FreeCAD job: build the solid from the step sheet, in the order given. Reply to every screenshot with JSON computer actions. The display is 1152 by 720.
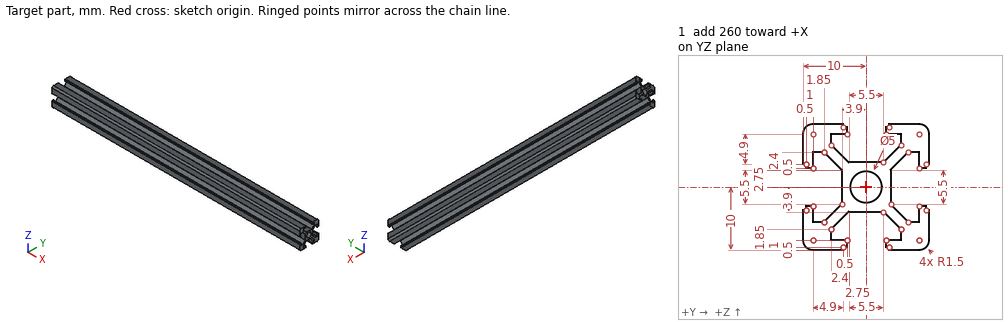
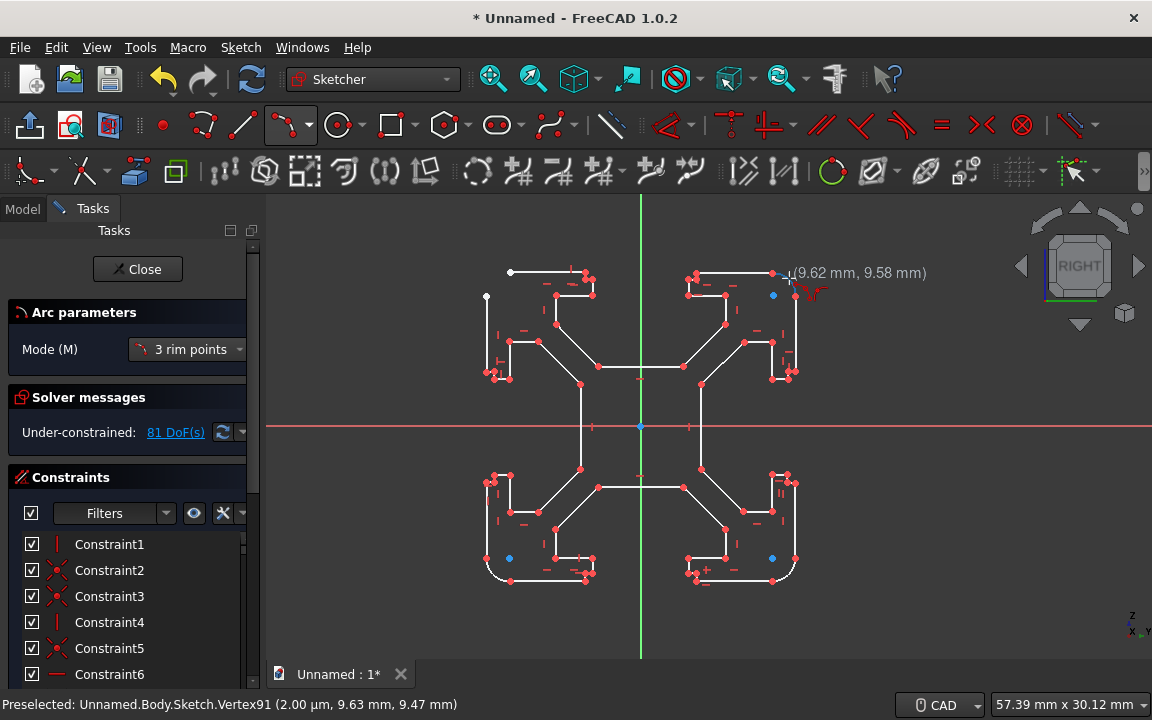
{"action": "left_click", "coordinate": [510, 272]}
{"action": "left_click", "coordinate": [487, 296]}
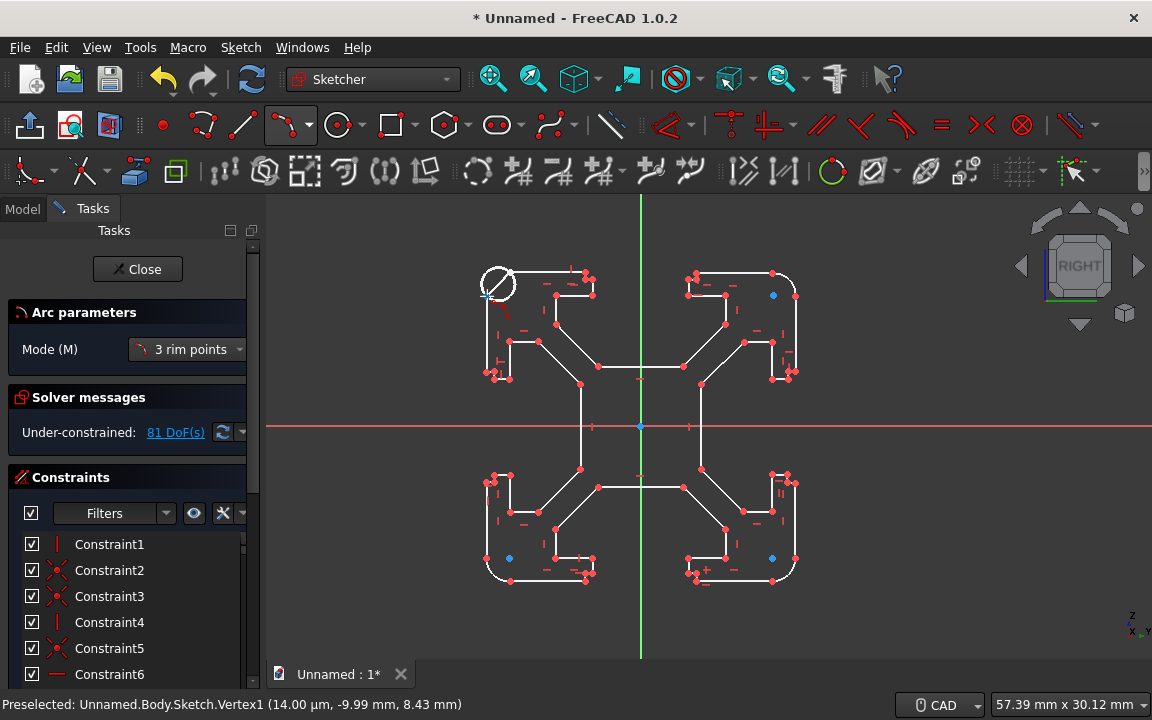
{"action": "scroll", "coordinate": [493, 279], "scroll_direction": "up", "scroll_amount": 5}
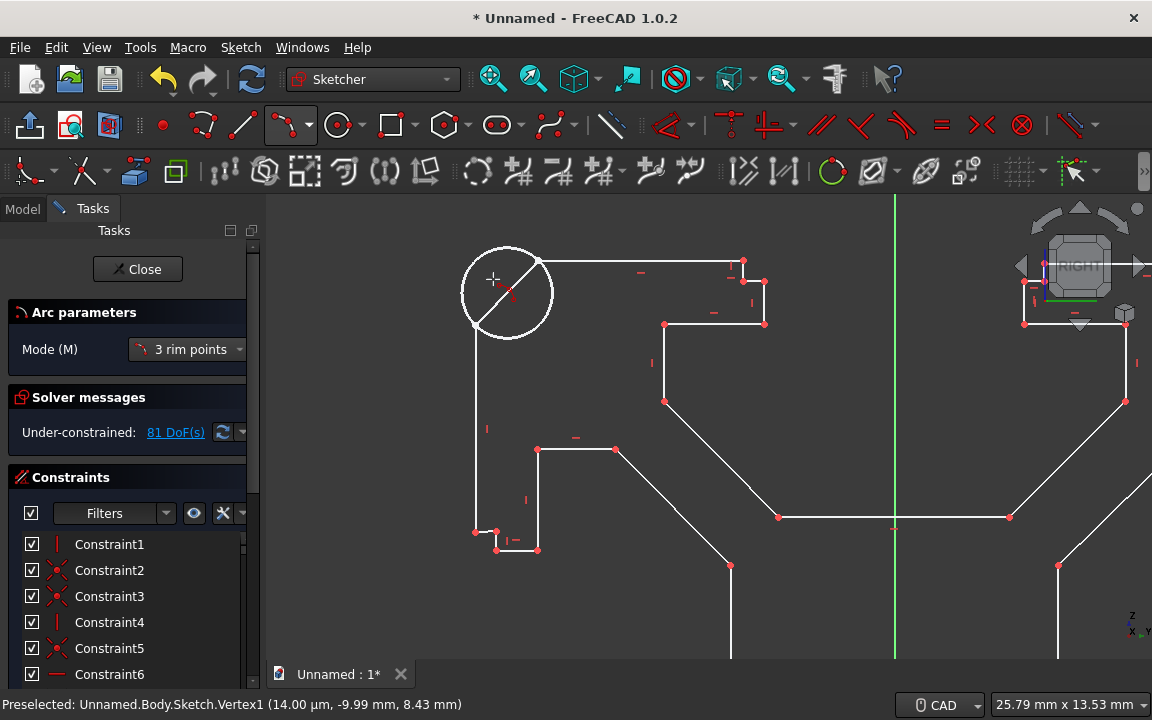
{"action": "left_click", "coordinate": [493, 278]}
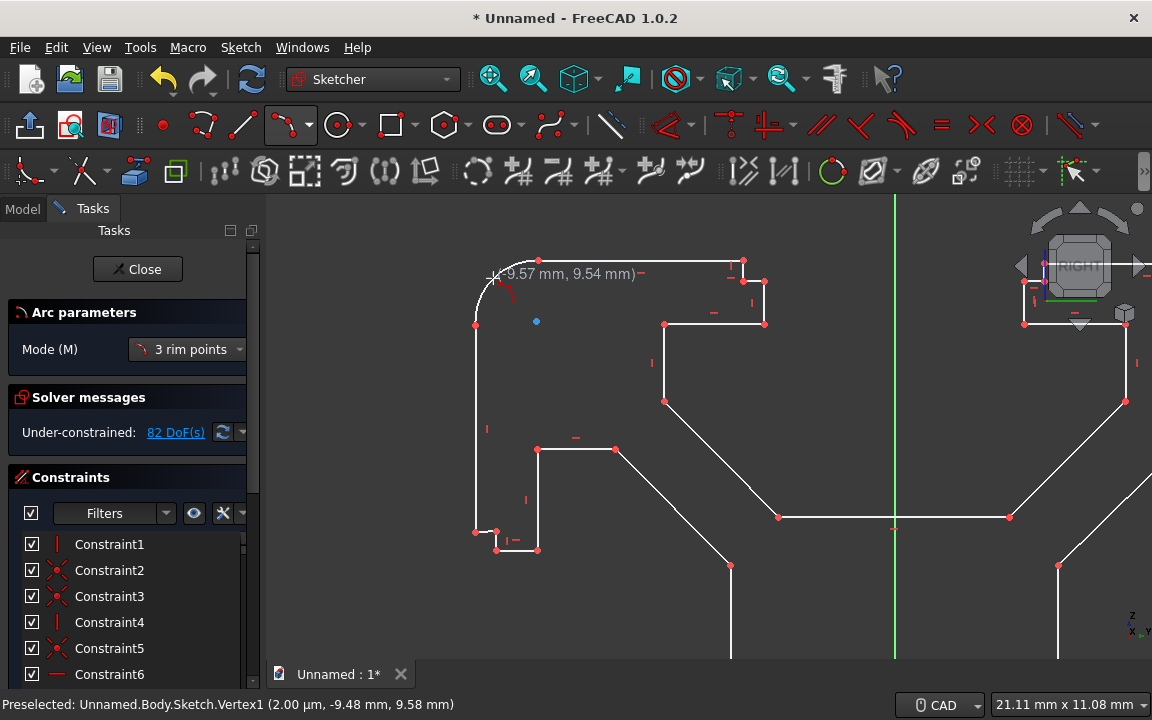
{"action": "left_click", "coordinate": [338, 126]}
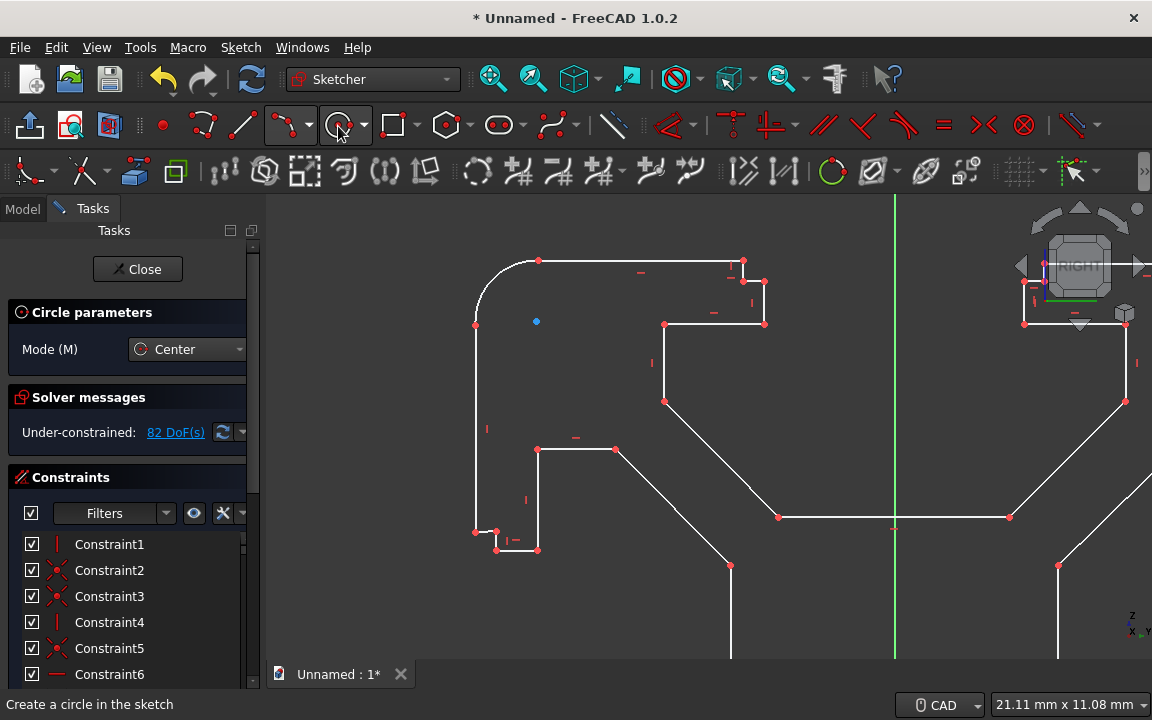
{"action": "scroll", "coordinate": [493, 279], "scroll_direction": "down", "scroll_amount": 5}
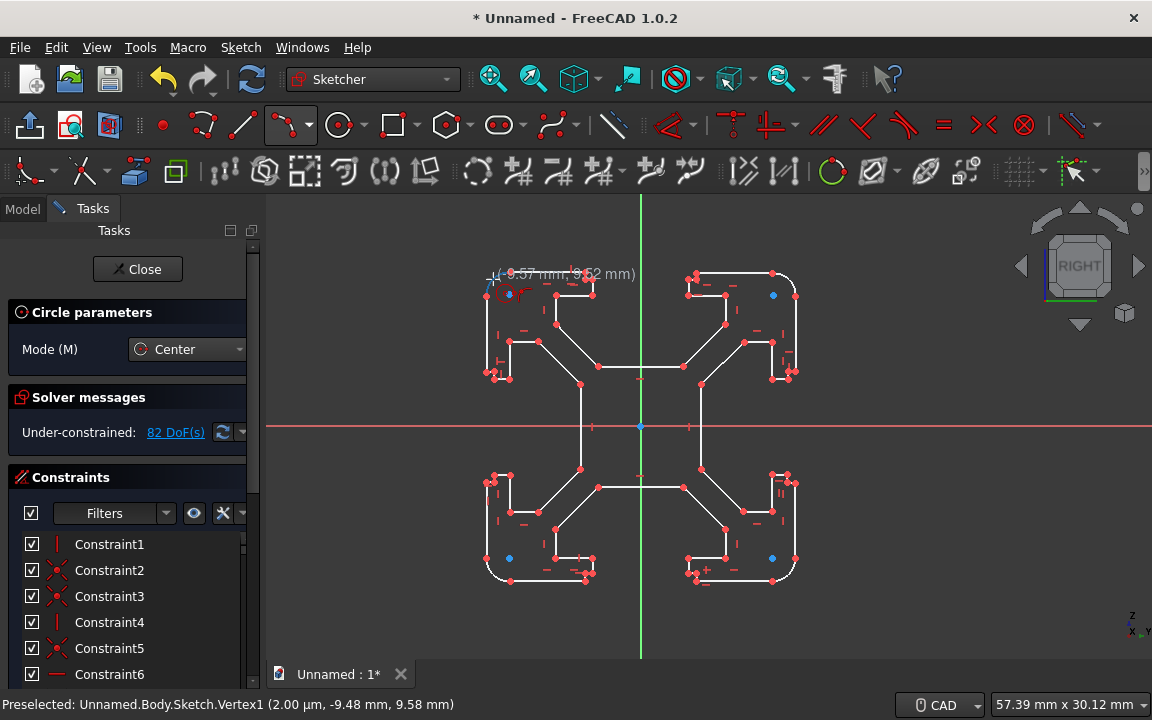
{"action": "left_click", "coordinate": [641, 426]}
{"action": "mouse_move", "coordinate": [668, 399]}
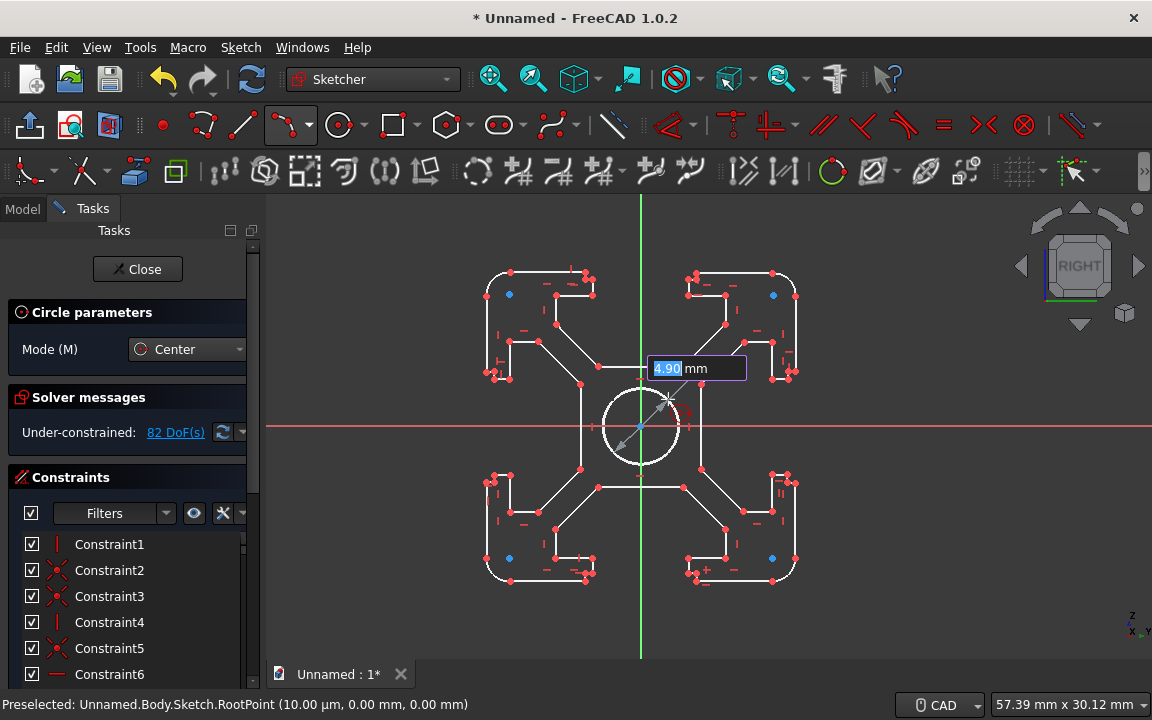
{"action": "type", "text": "5"}
{"action": "key", "text": "Return"}
{"action": "key", "text": "Escape"}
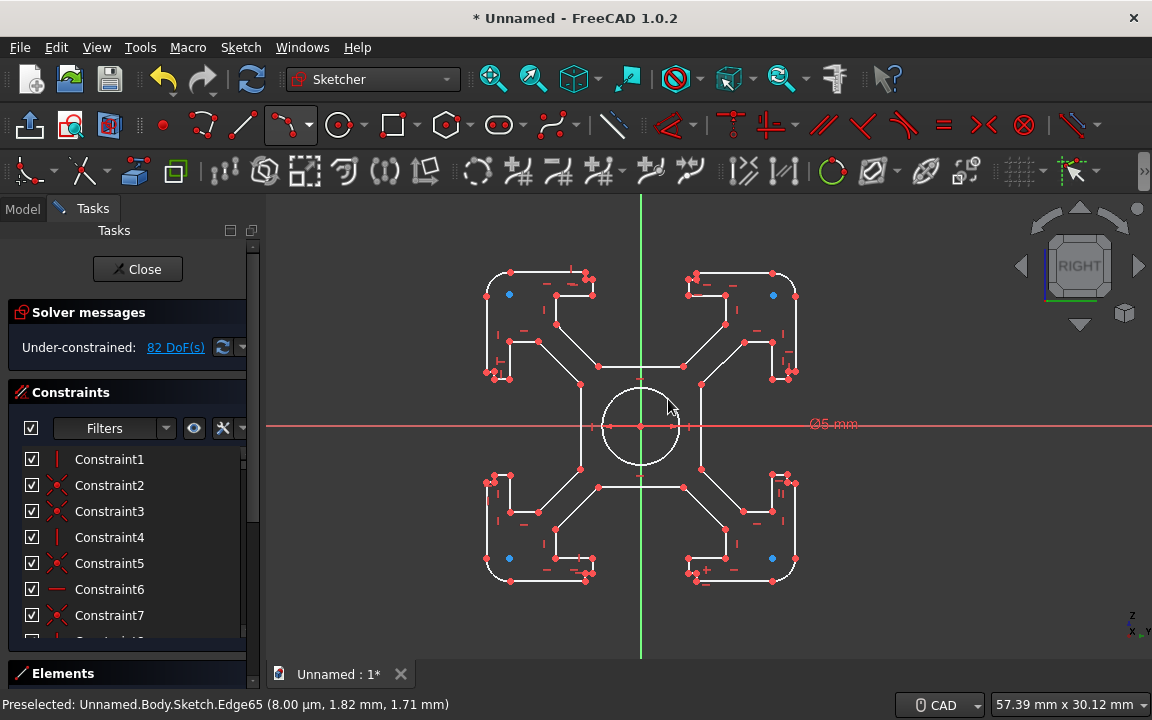
{"action": "left_click", "coordinate": [487, 319]}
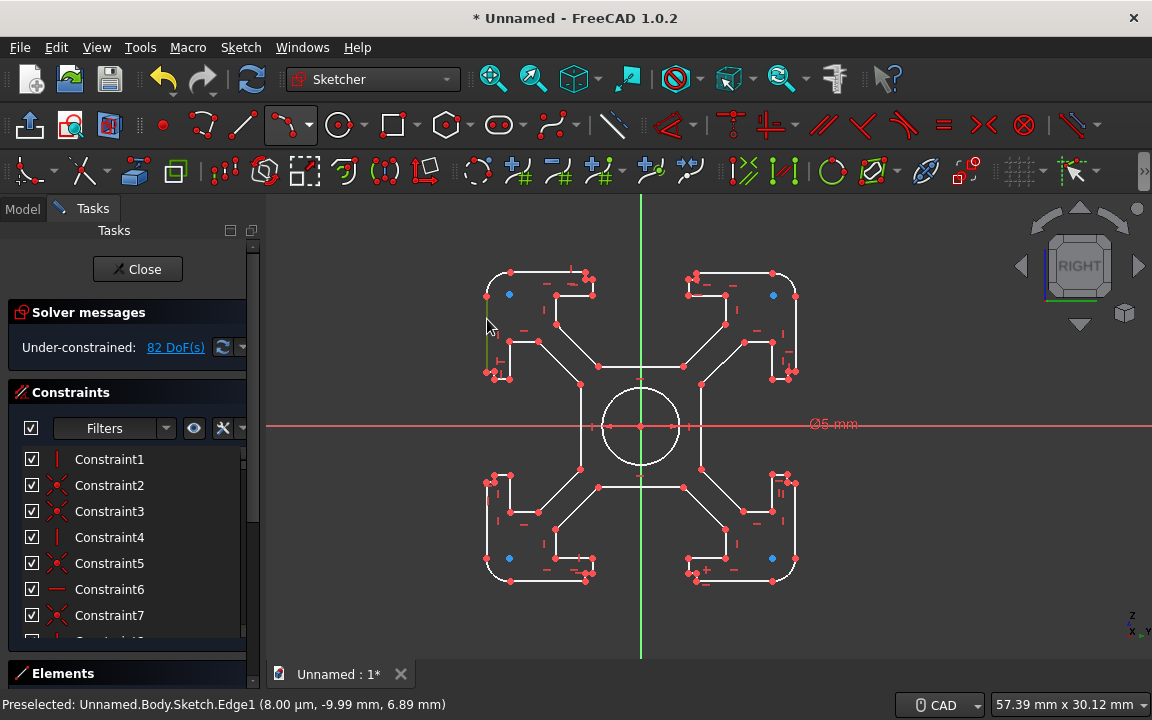
{"action": "scroll", "coordinate": [499, 275], "scroll_direction": "up", "scroll_amount": 2}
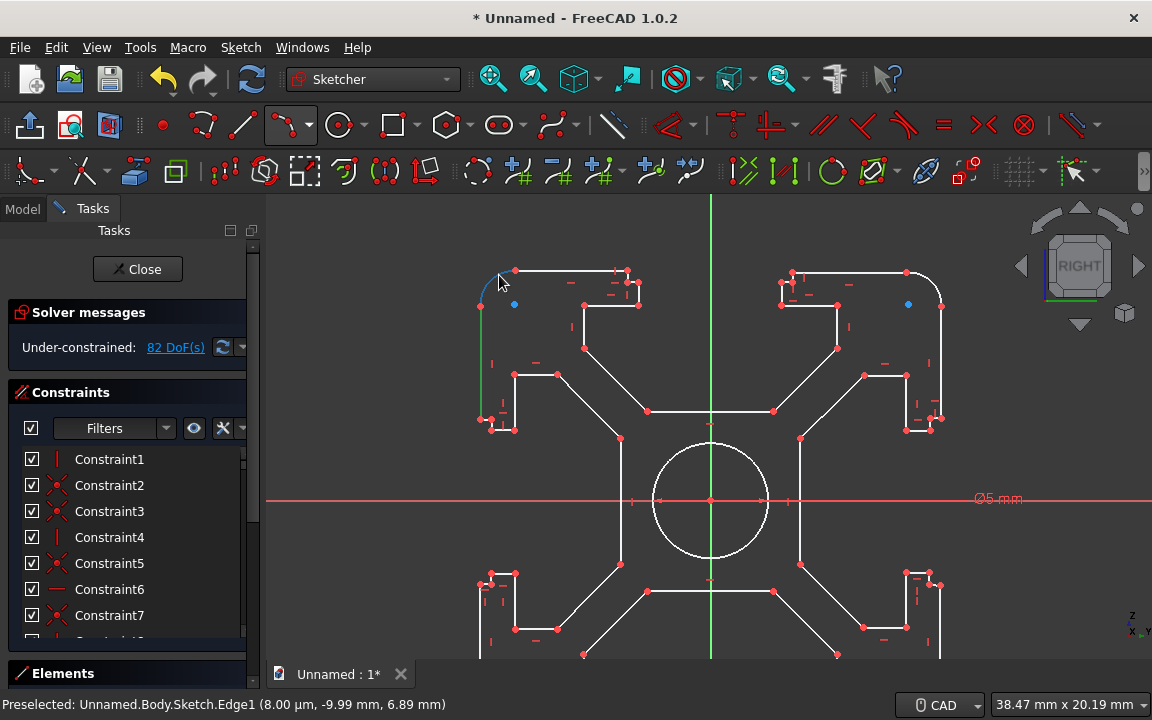
{"action": "left_click", "coordinate": [499, 275]}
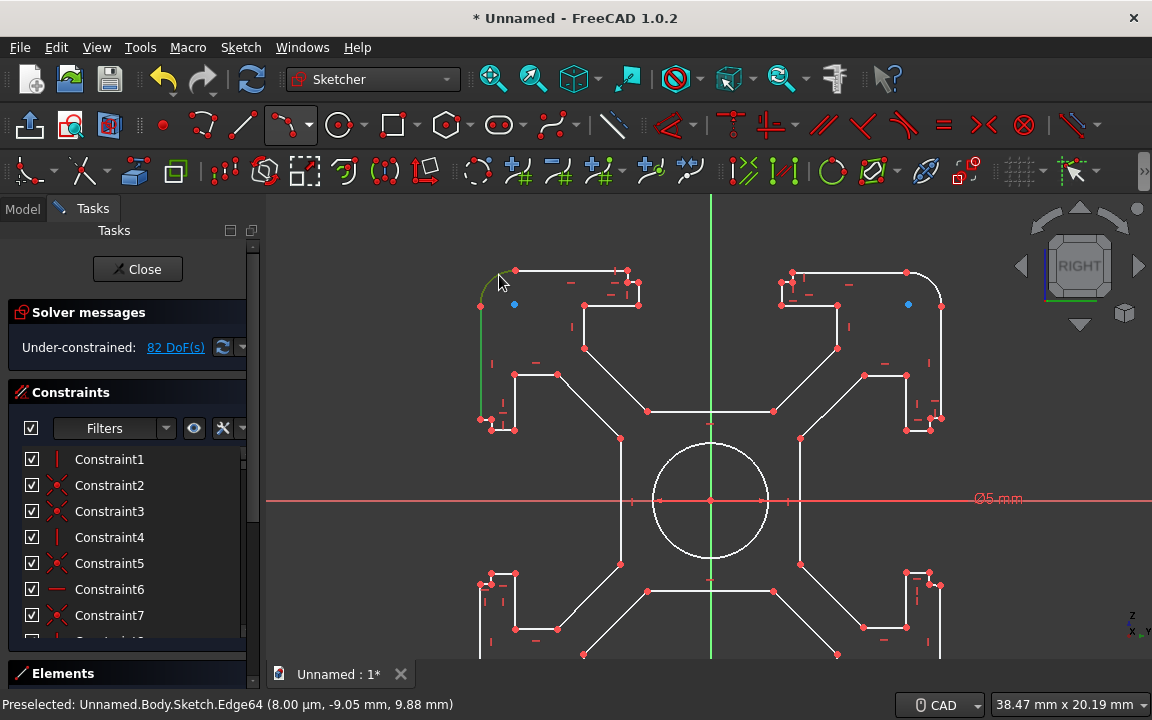
{"action": "left_click", "coordinate": [904, 126]}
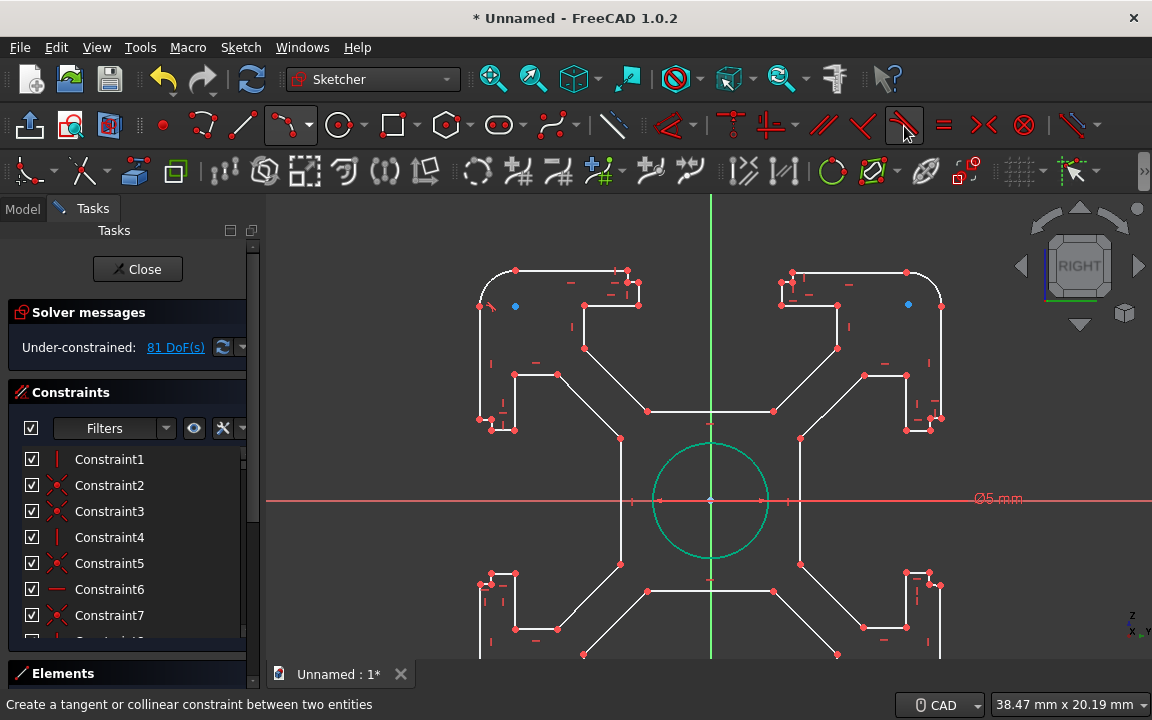
{"action": "left_click", "coordinate": [480, 618]}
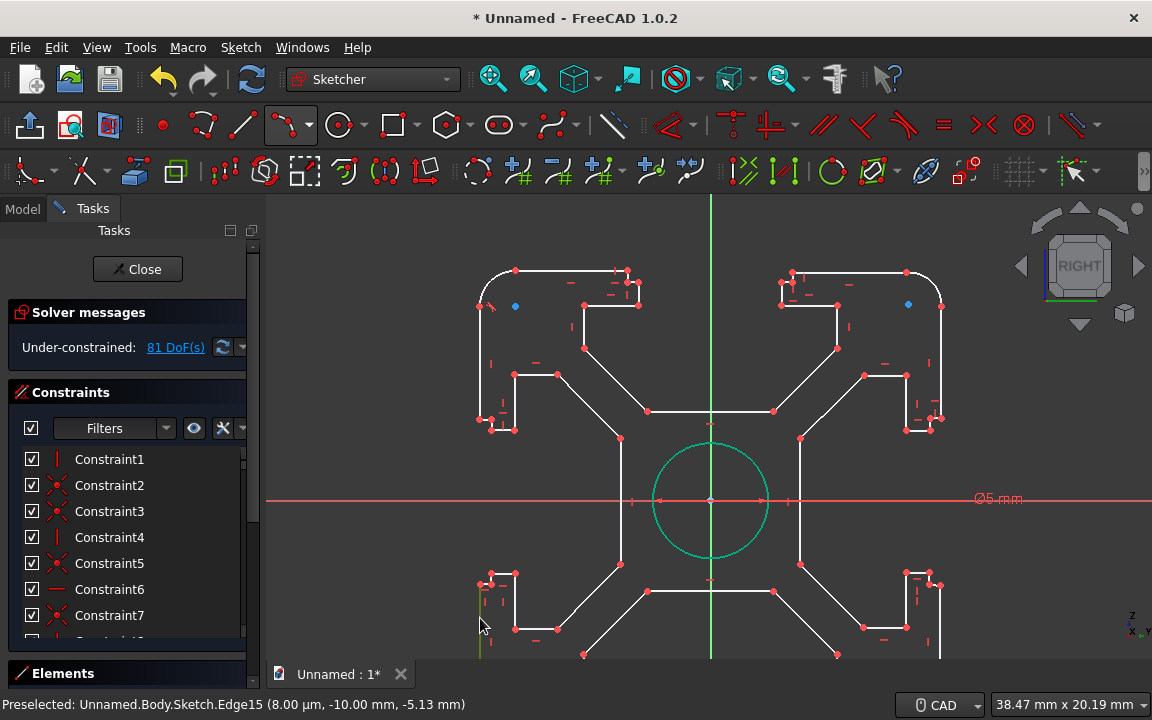
{"action": "scroll", "coordinate": [498, 276], "scroll_direction": "down", "scroll_amount": 2}